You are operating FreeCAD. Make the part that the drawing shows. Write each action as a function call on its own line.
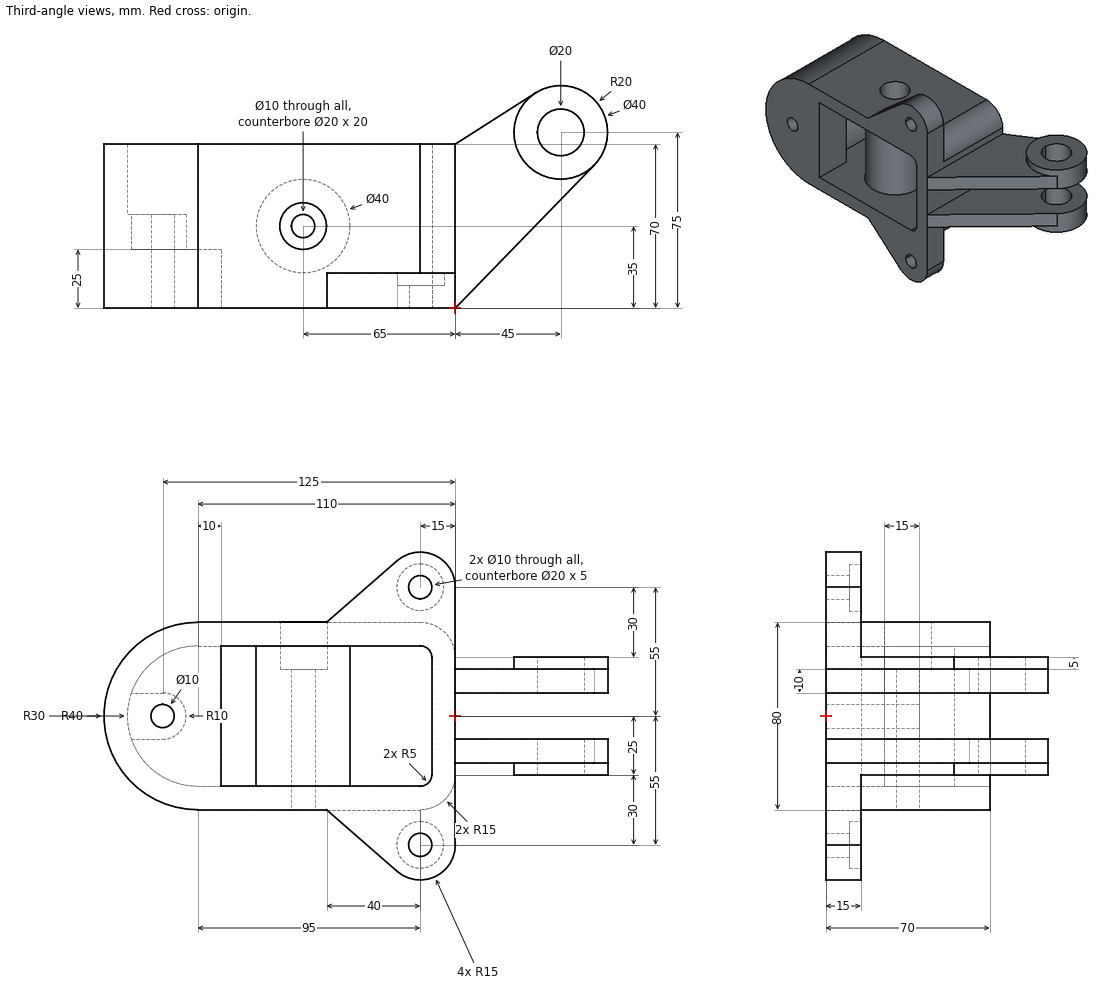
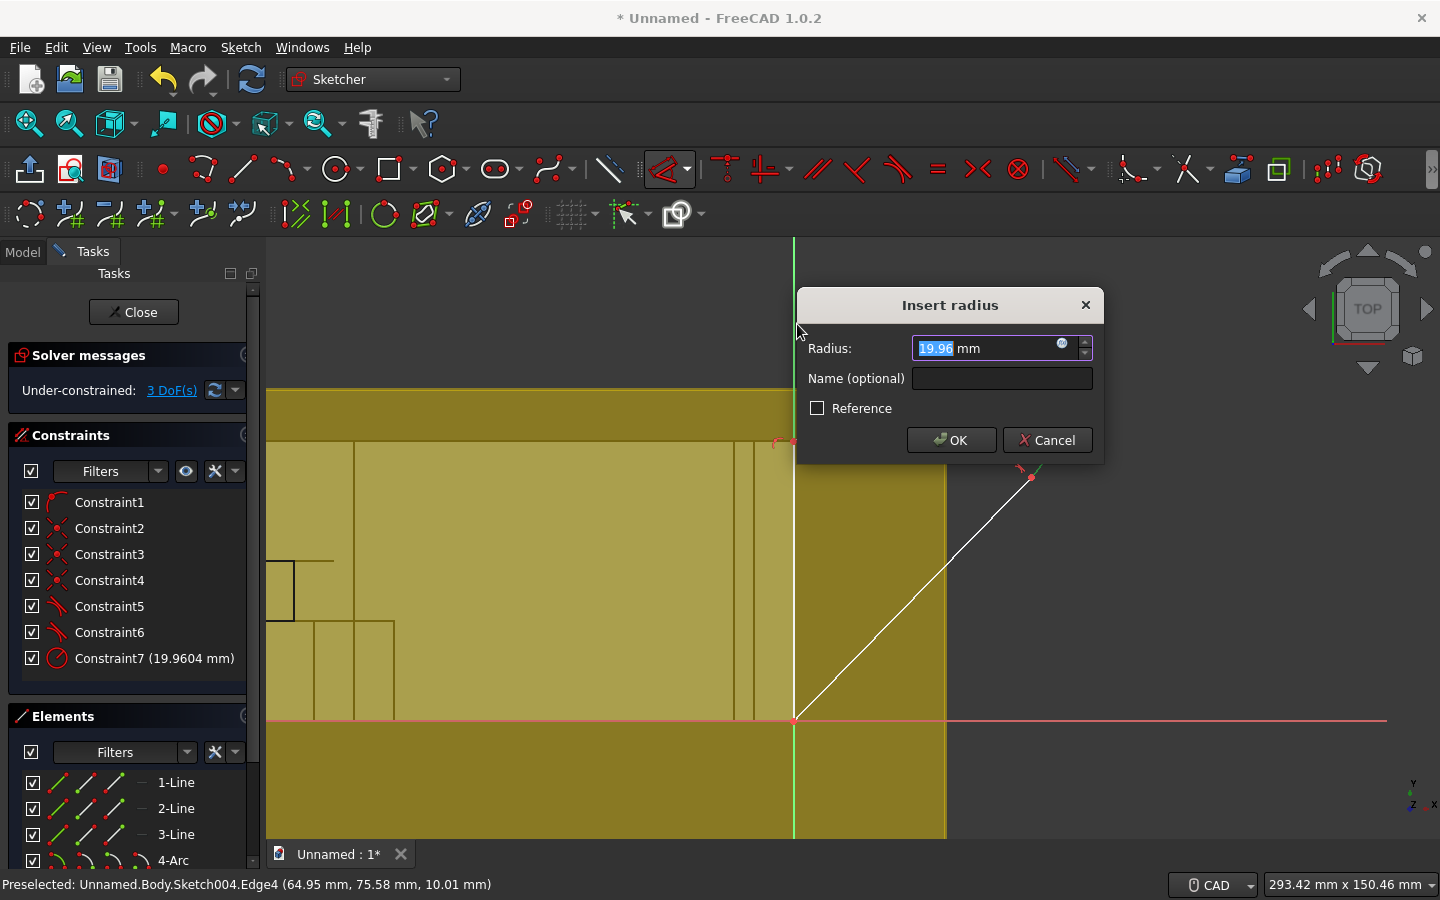
text(20)
key(Return)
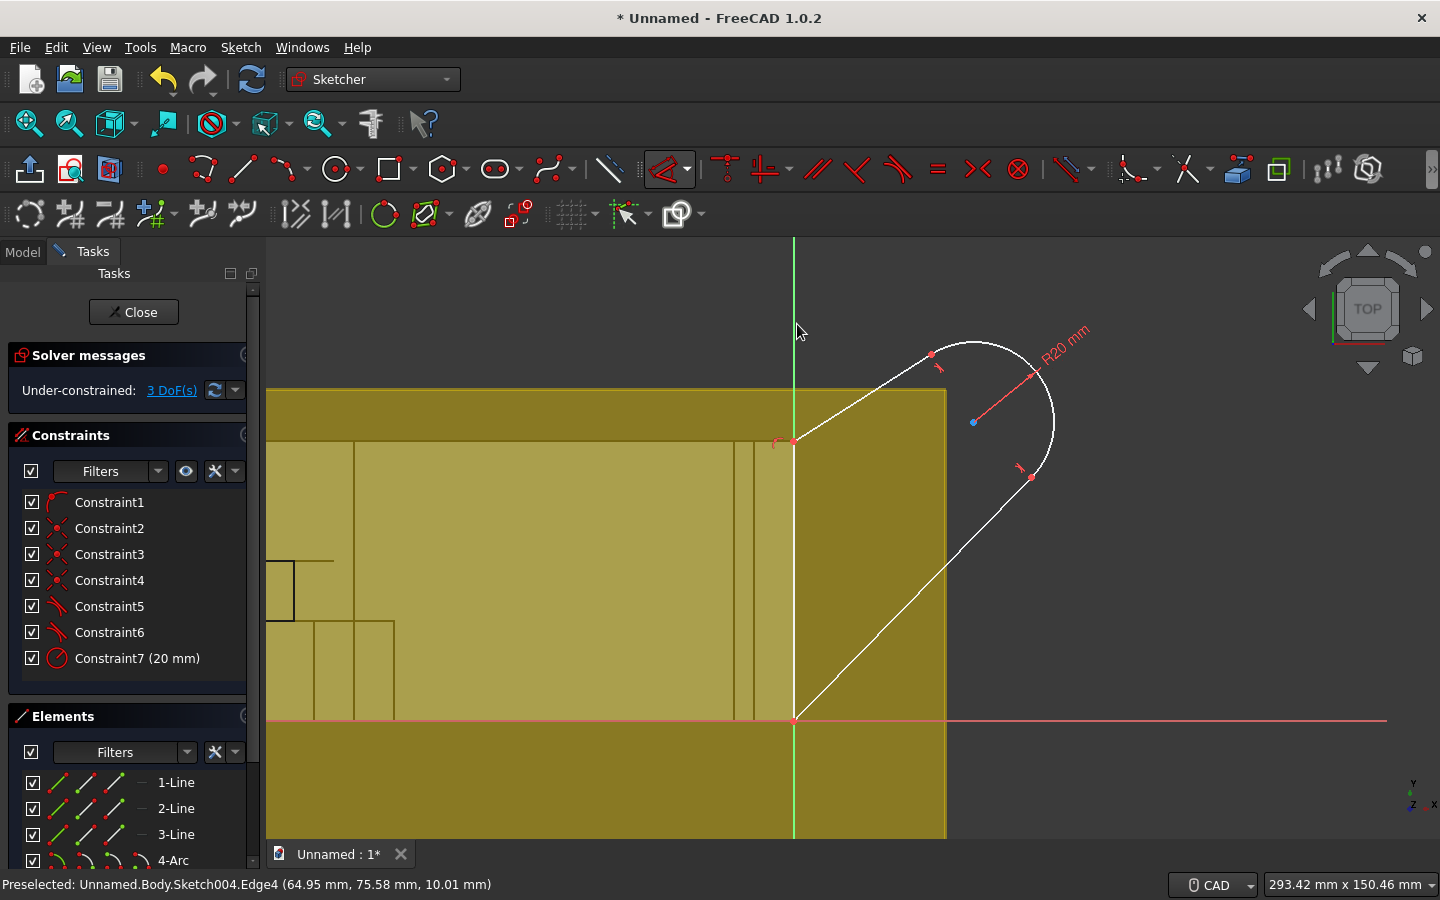
click(794, 526)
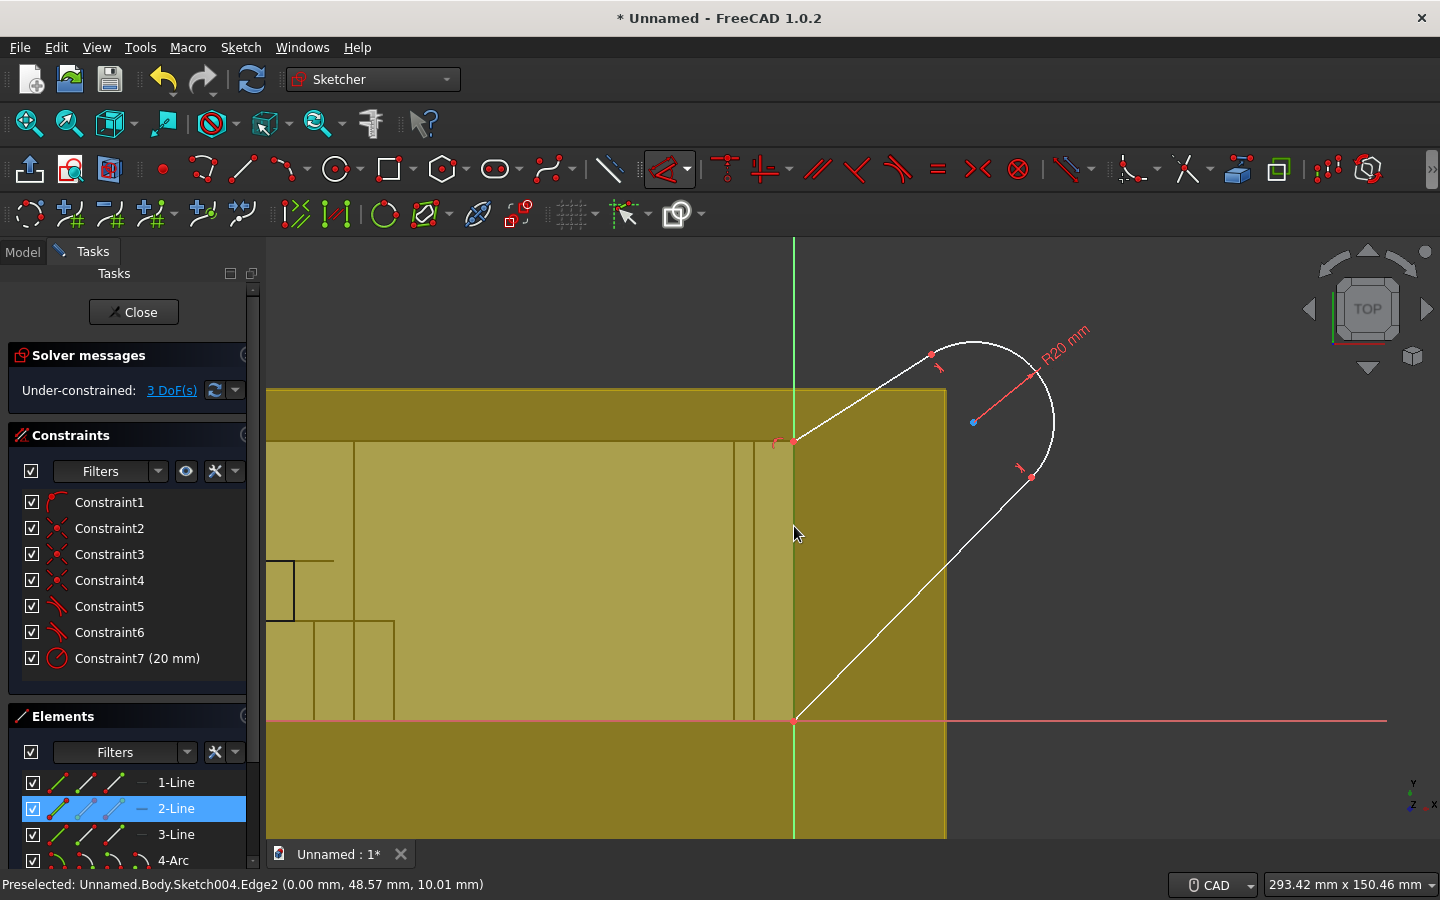
key(i)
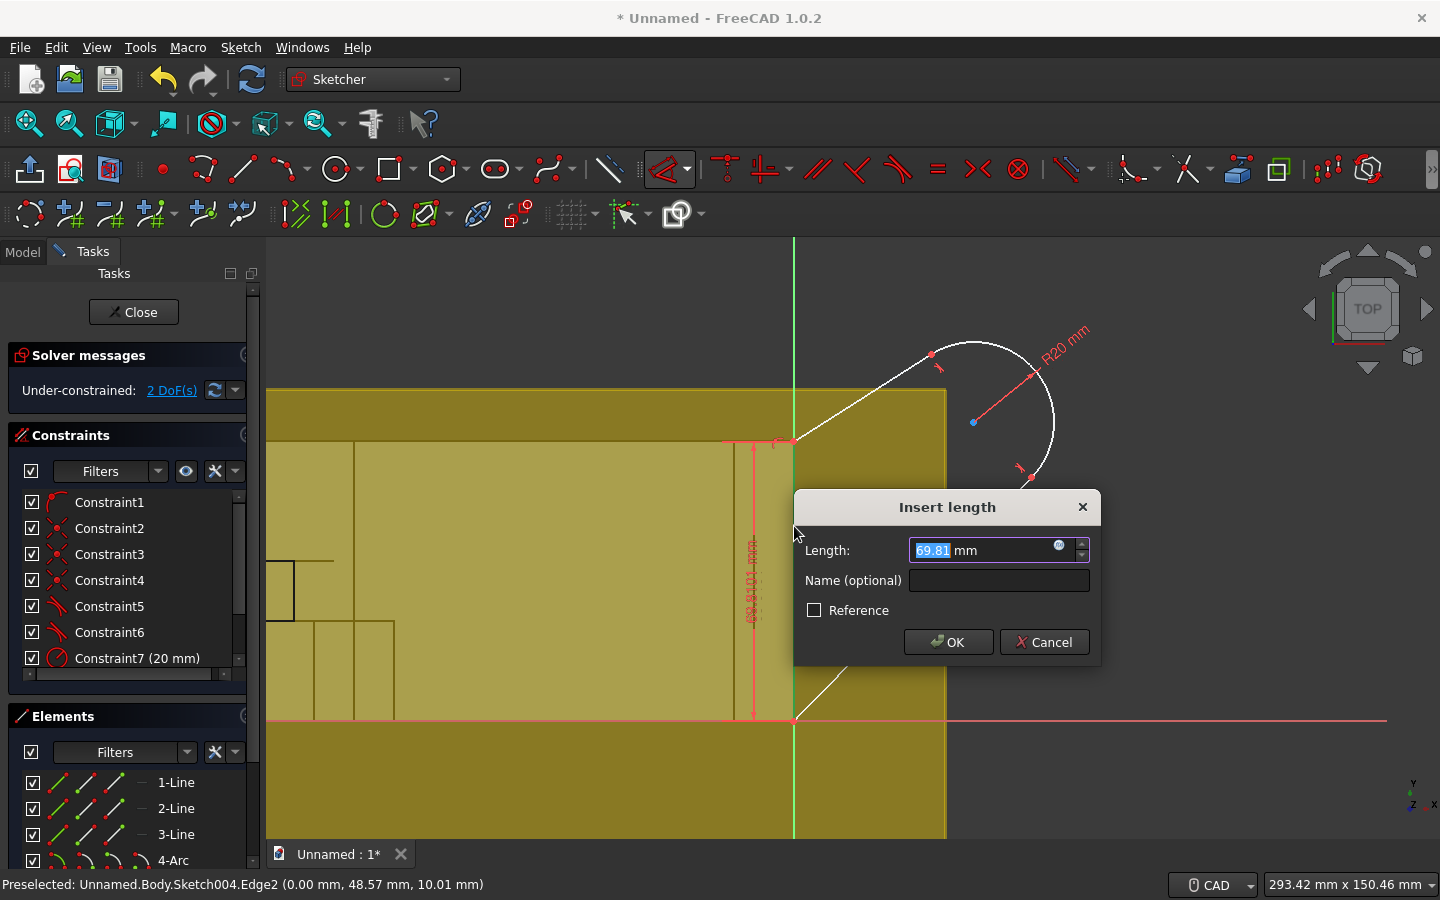
text(70)
key(Return)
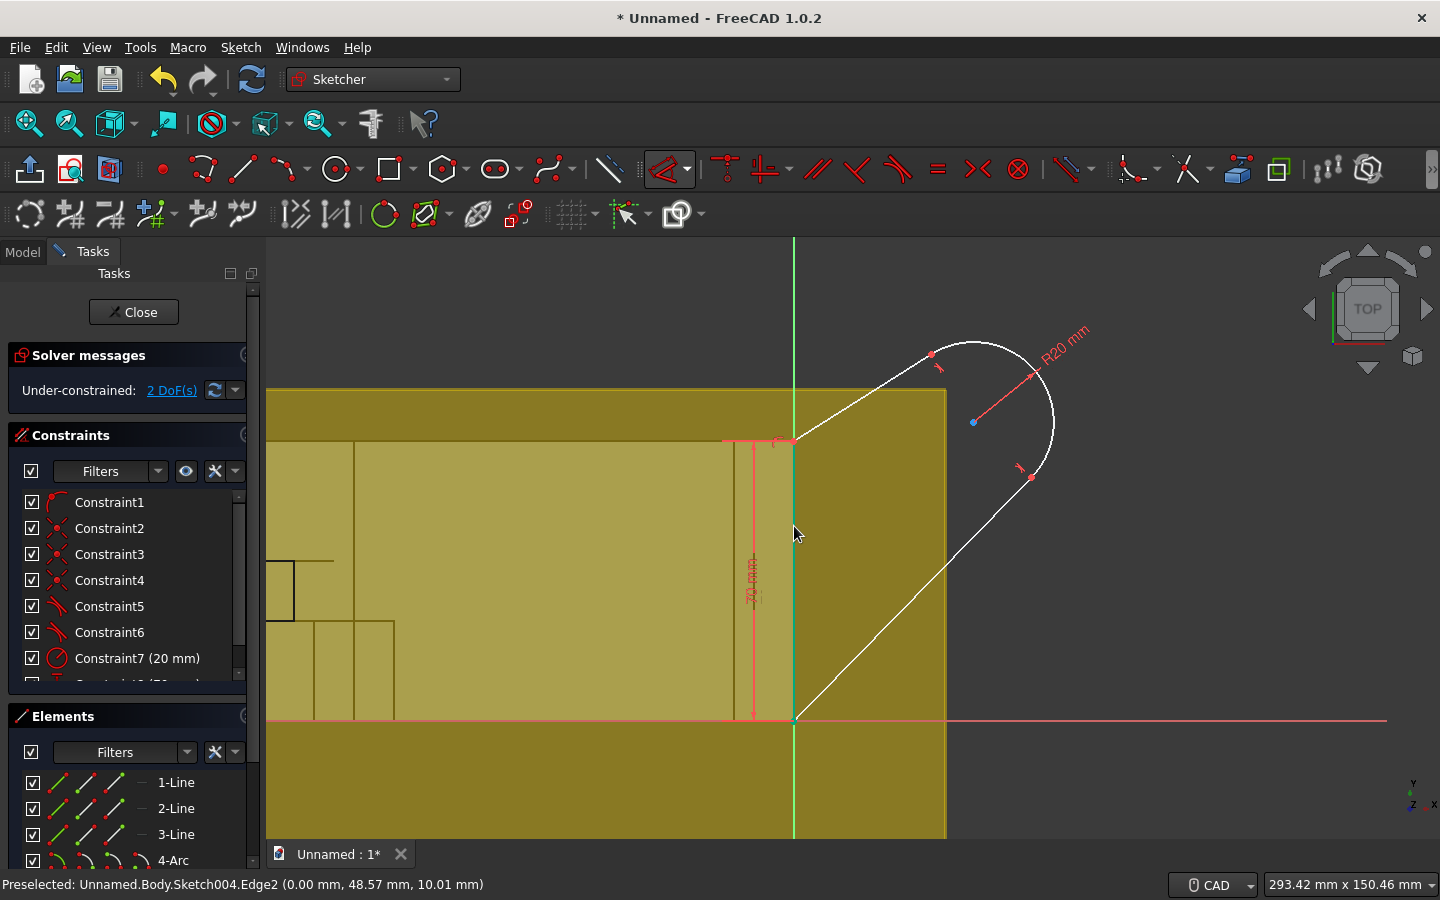
click(974, 422)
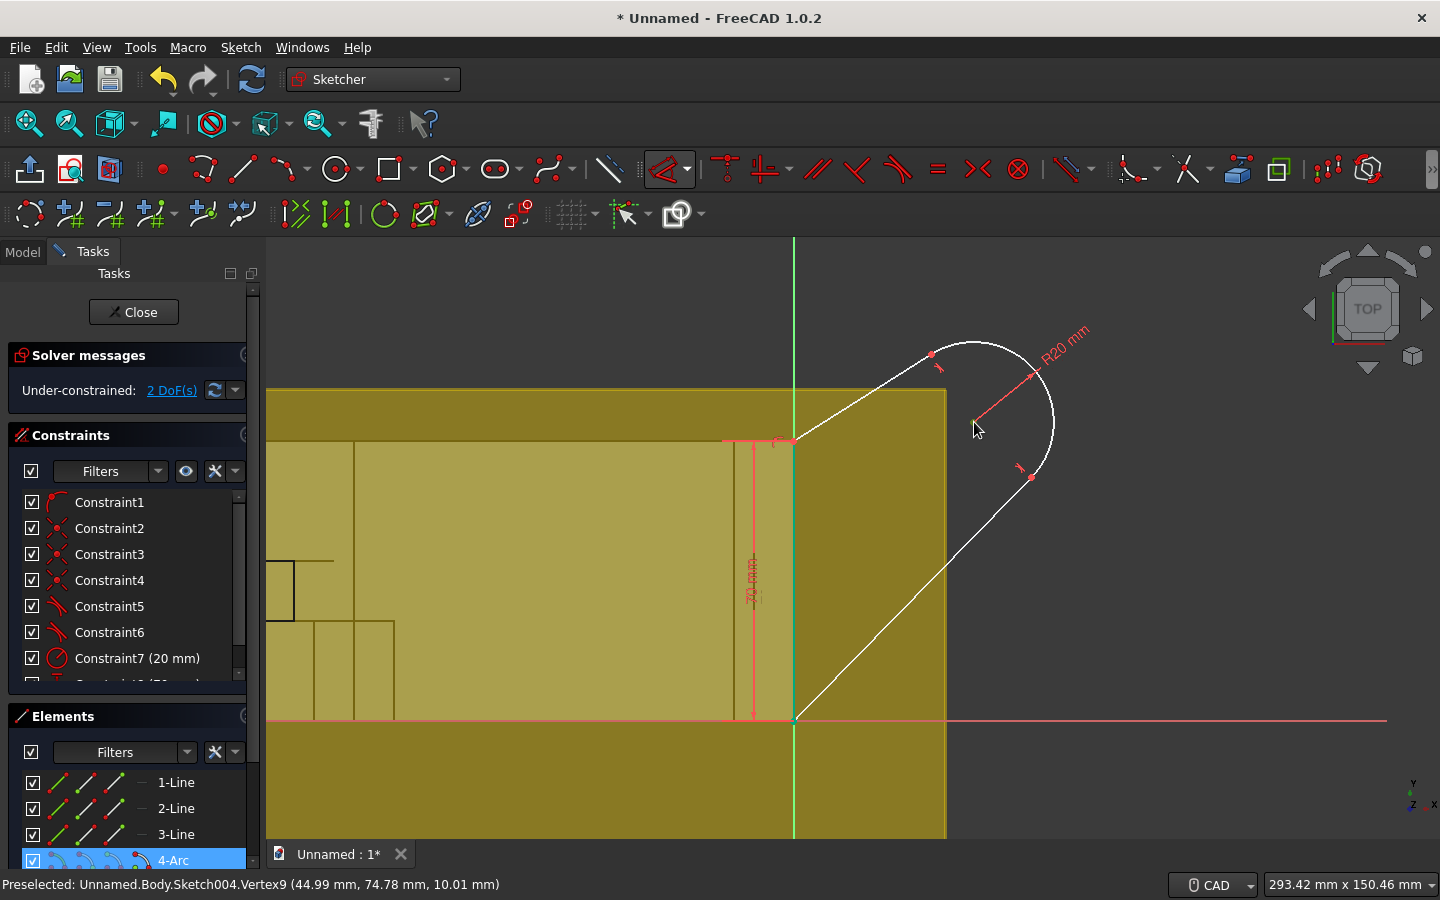
key(l)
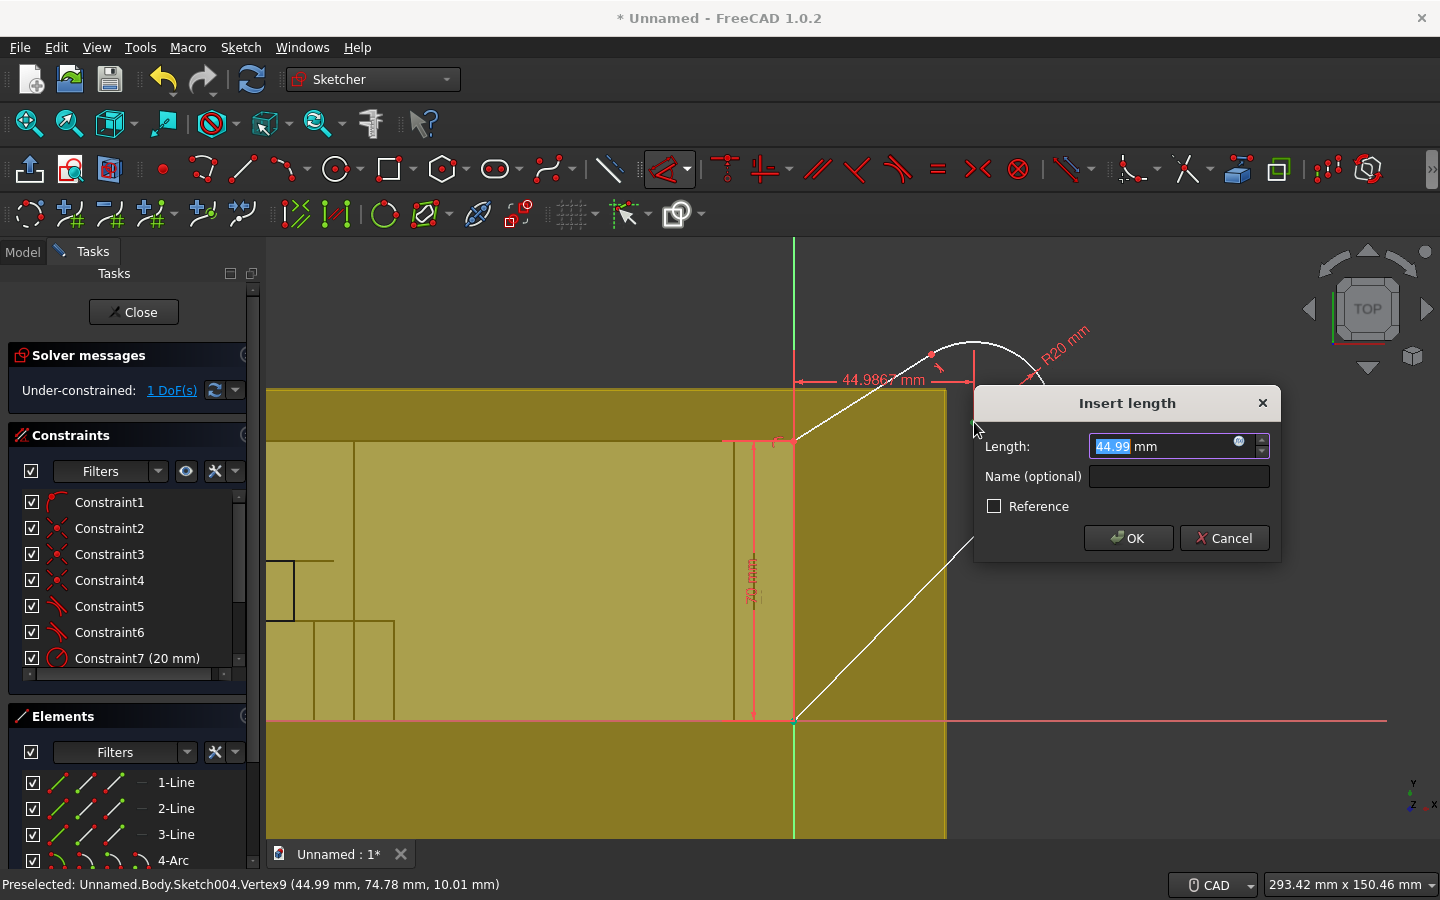
text(45)
key(Return)